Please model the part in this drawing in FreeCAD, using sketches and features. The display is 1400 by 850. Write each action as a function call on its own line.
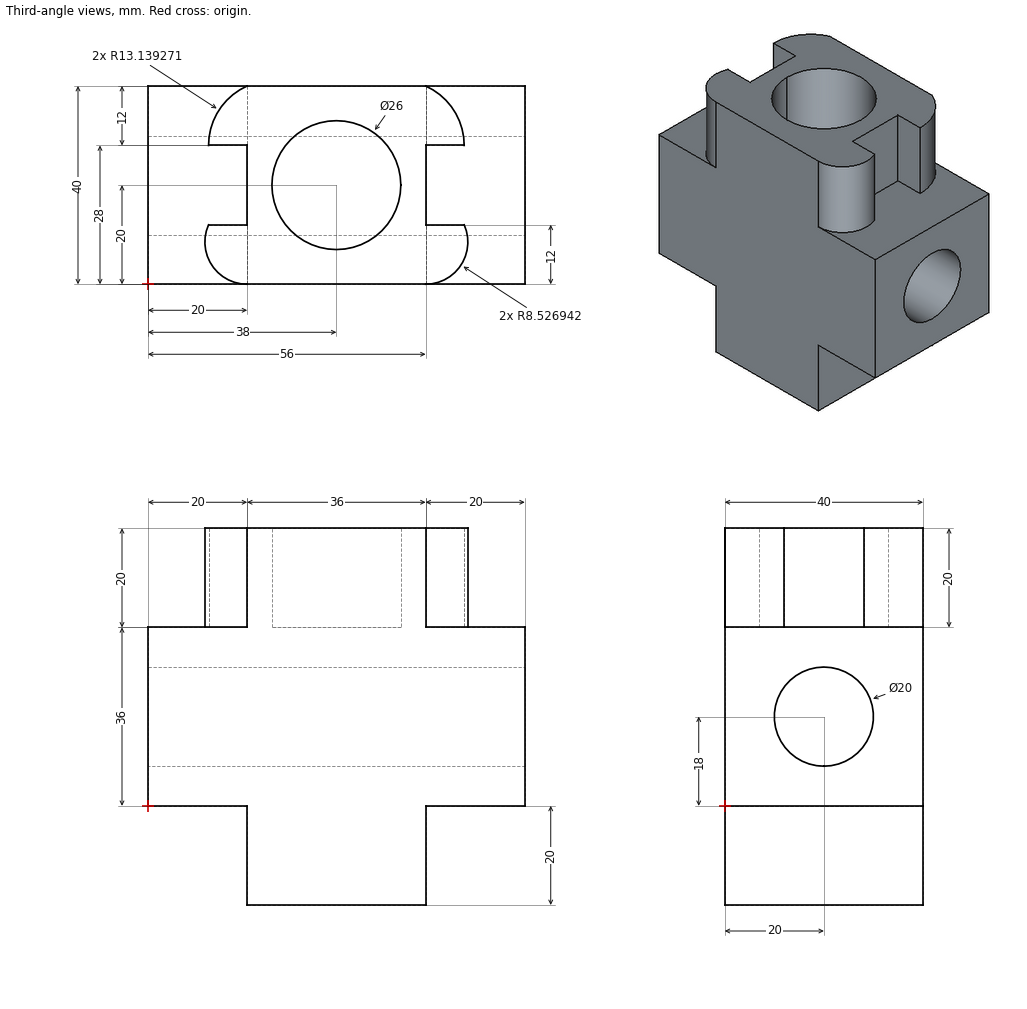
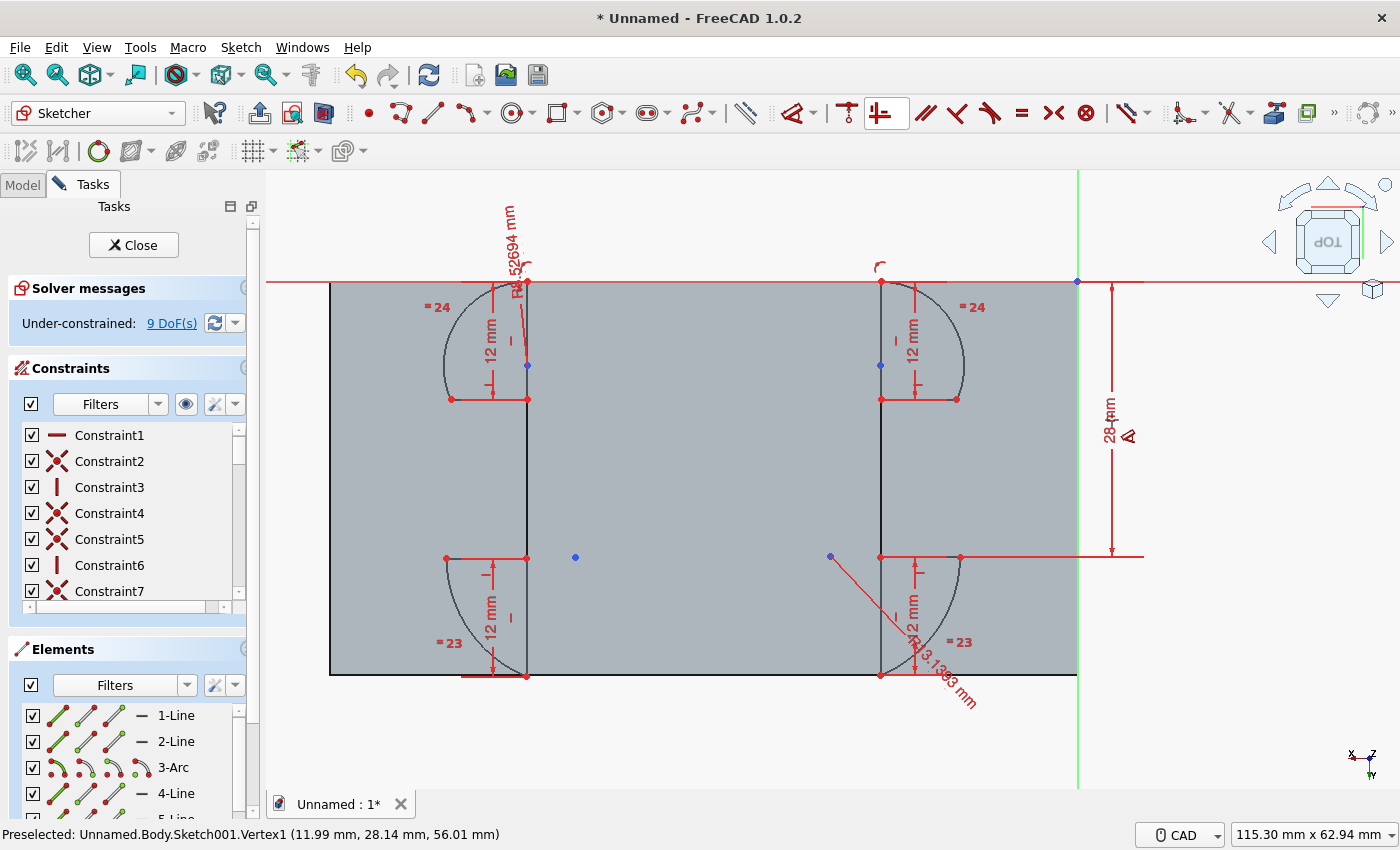
click(881, 557)
click(979, 248)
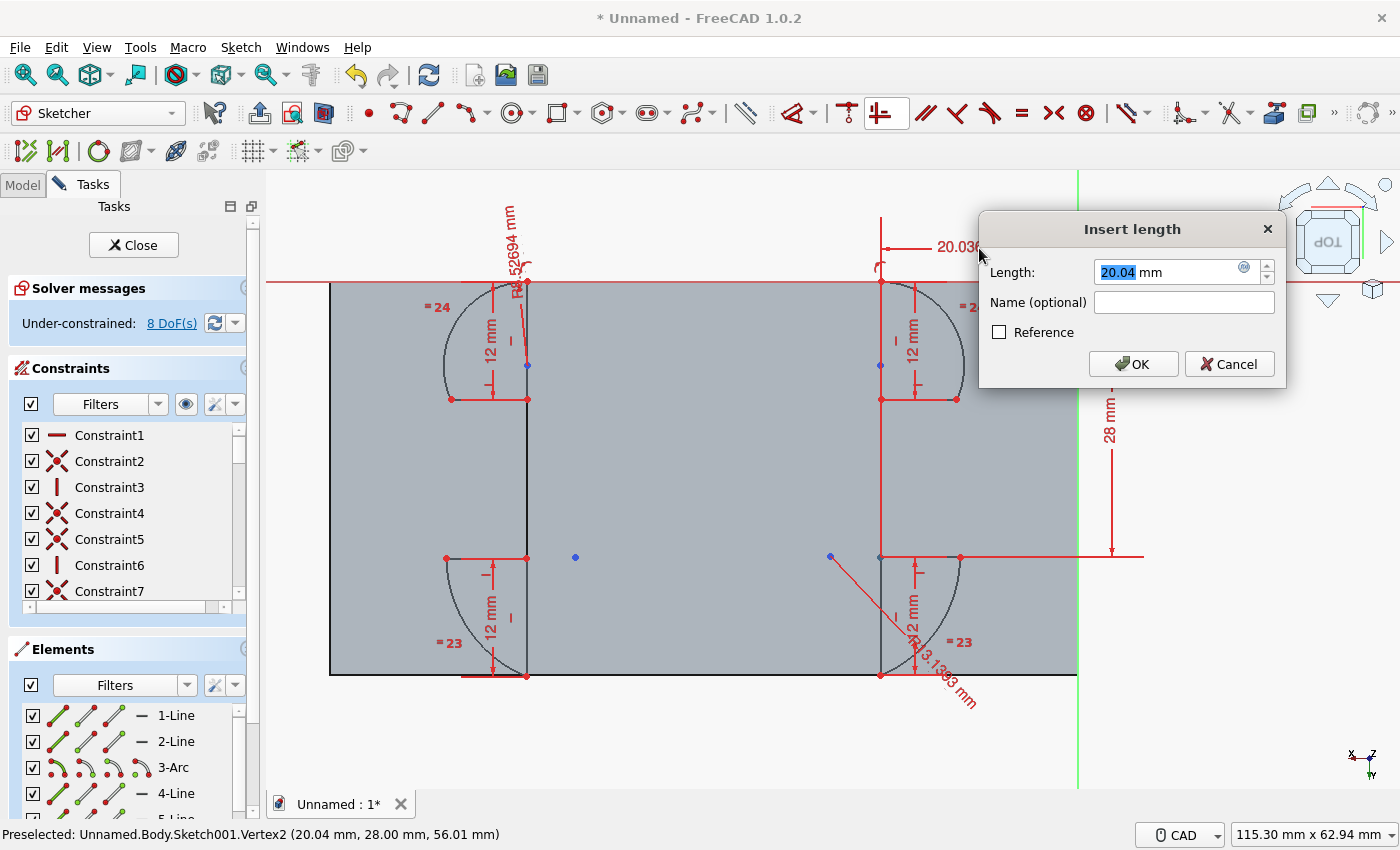
text(20)
key(Return)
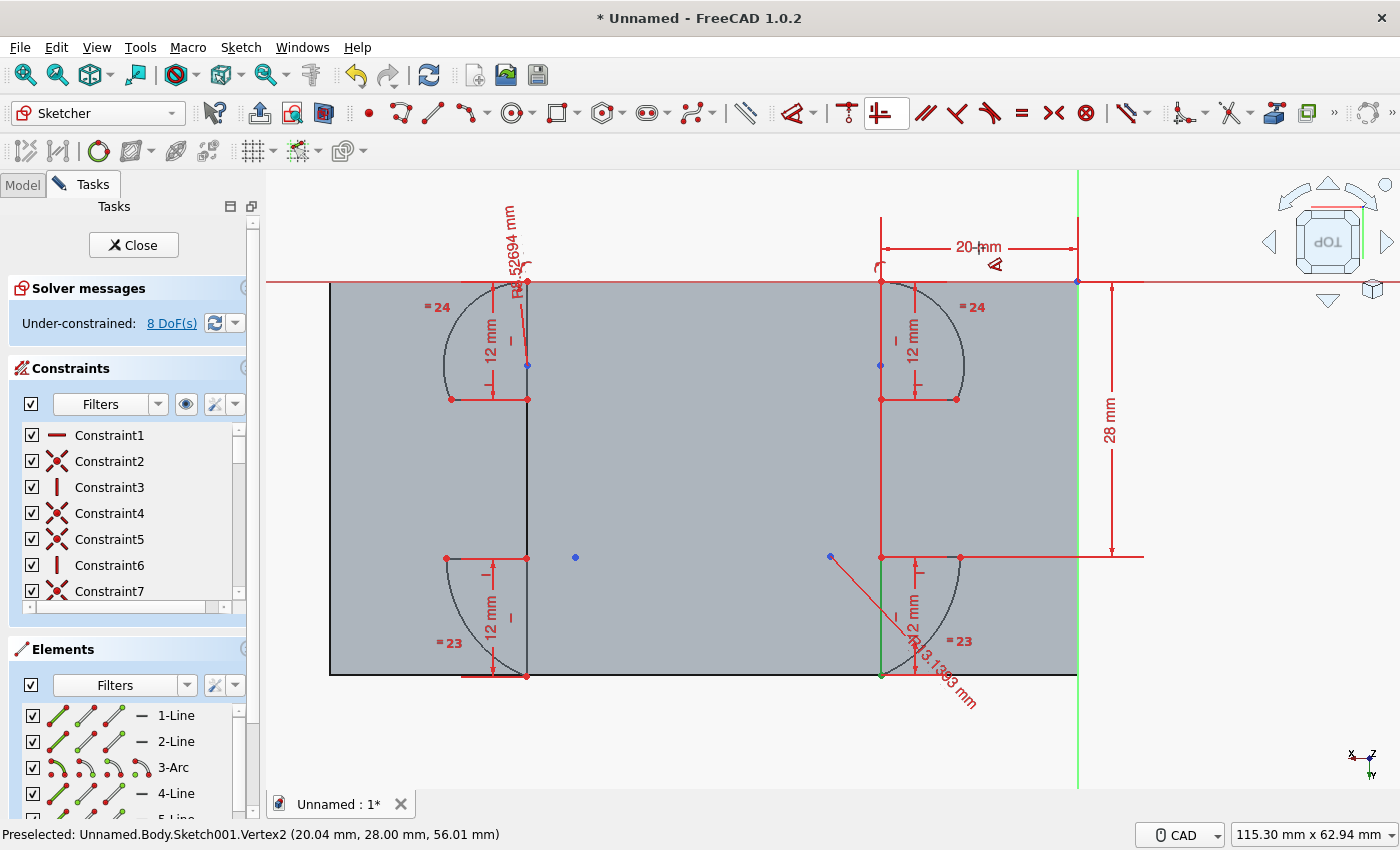
click(527, 677)
click(802, 711)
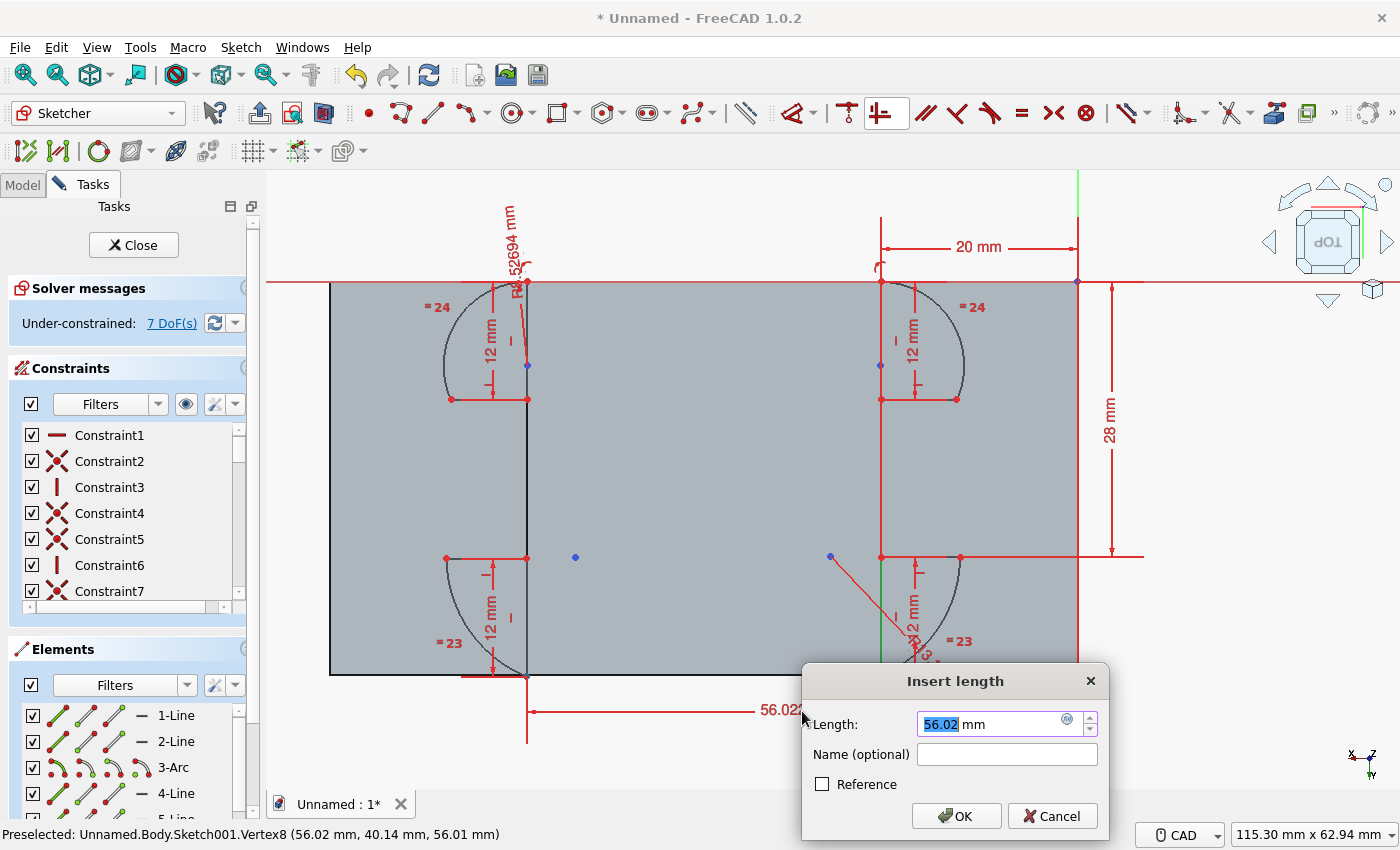
text(56)
key(Return)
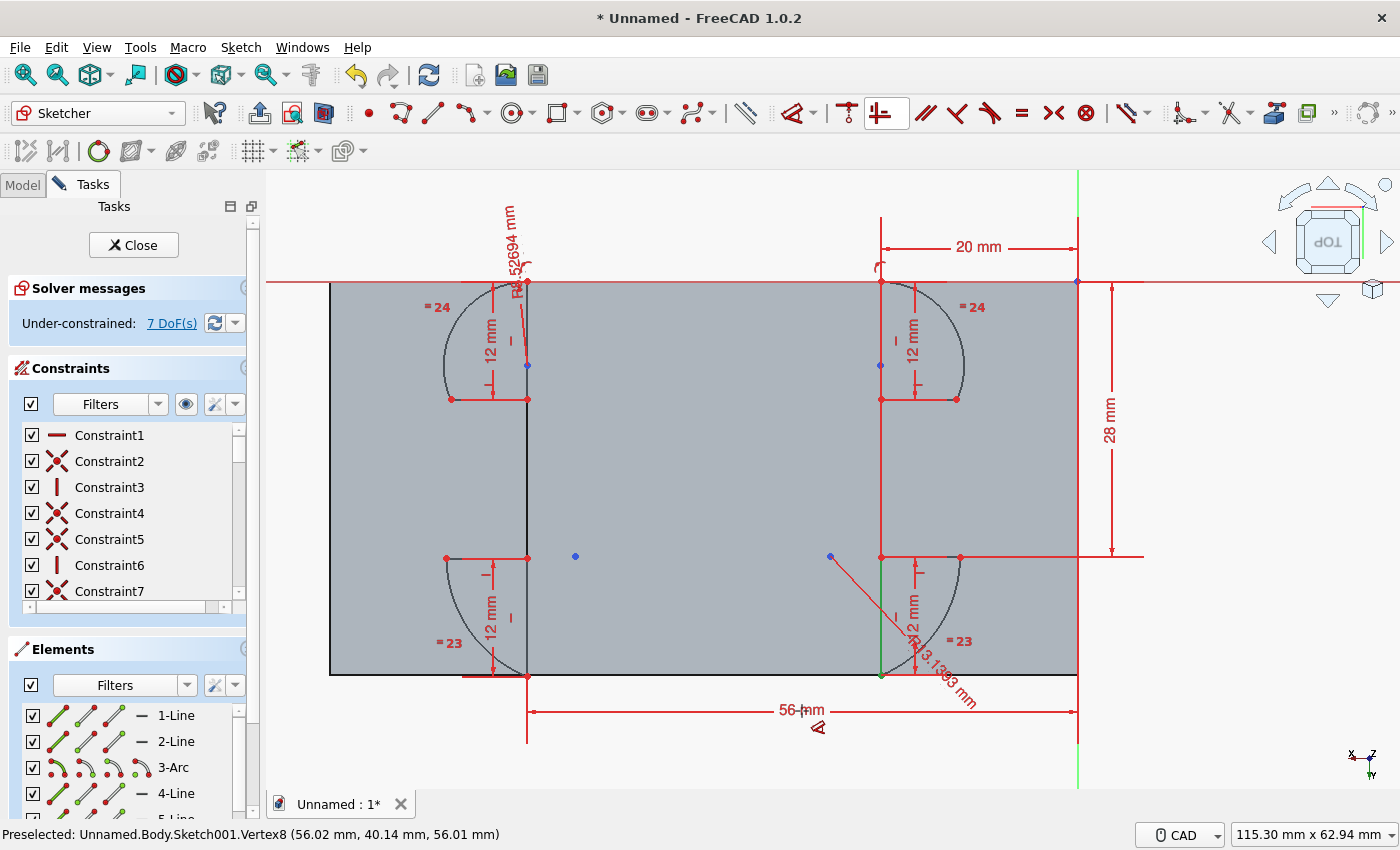
click(527, 677)
click(1112, 479)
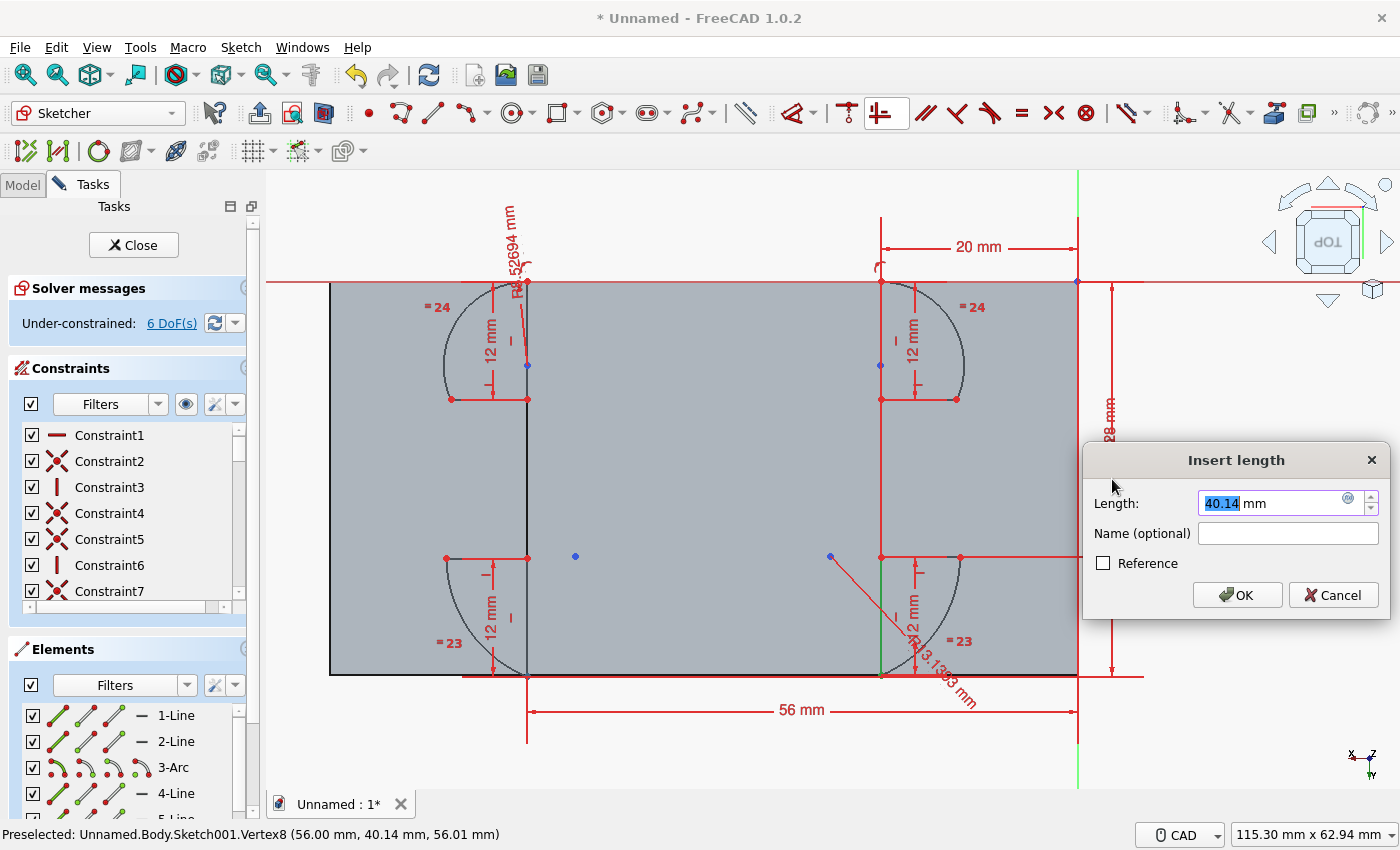
text(40)
key(Return)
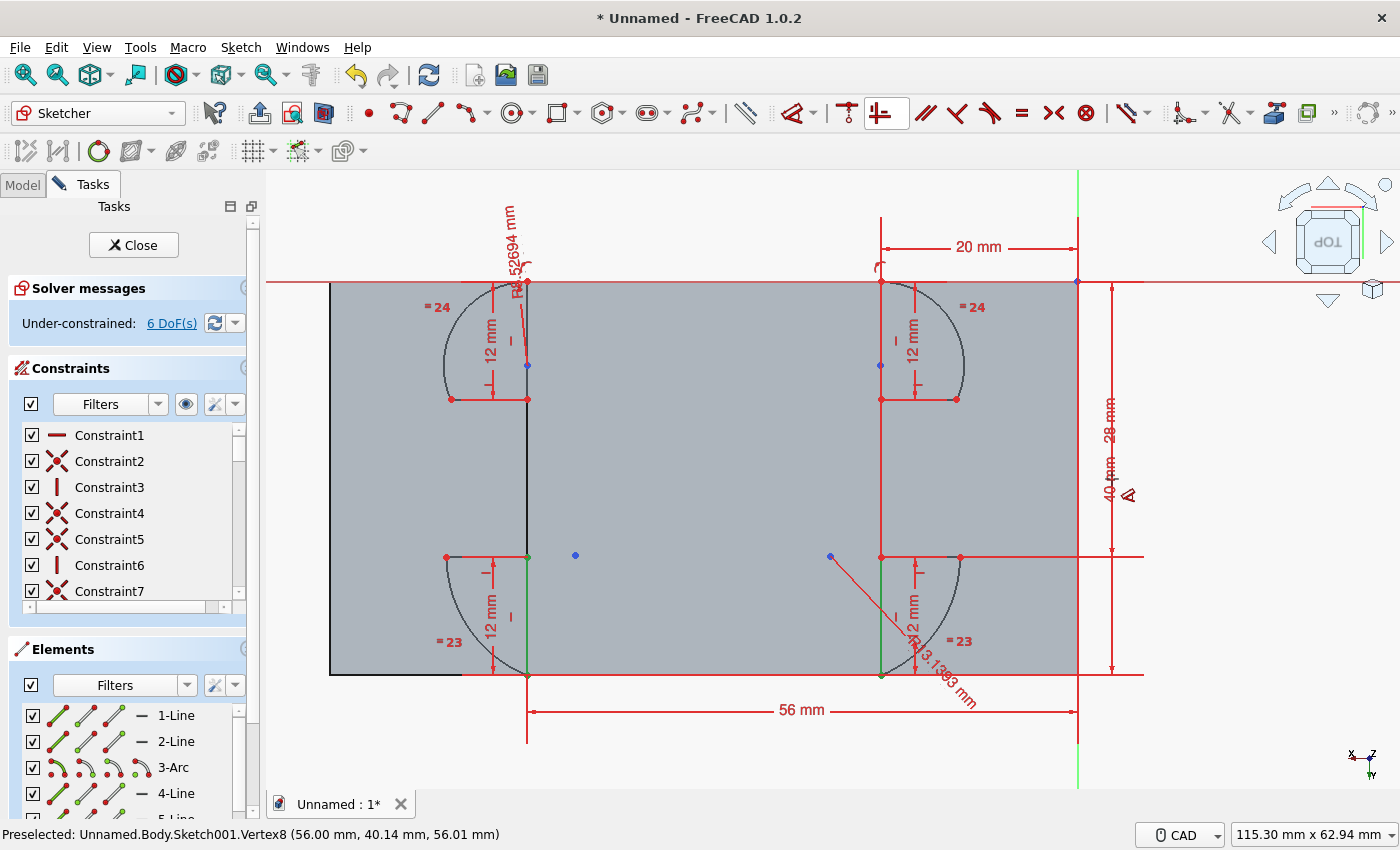
click(527, 400)
click(802, 248)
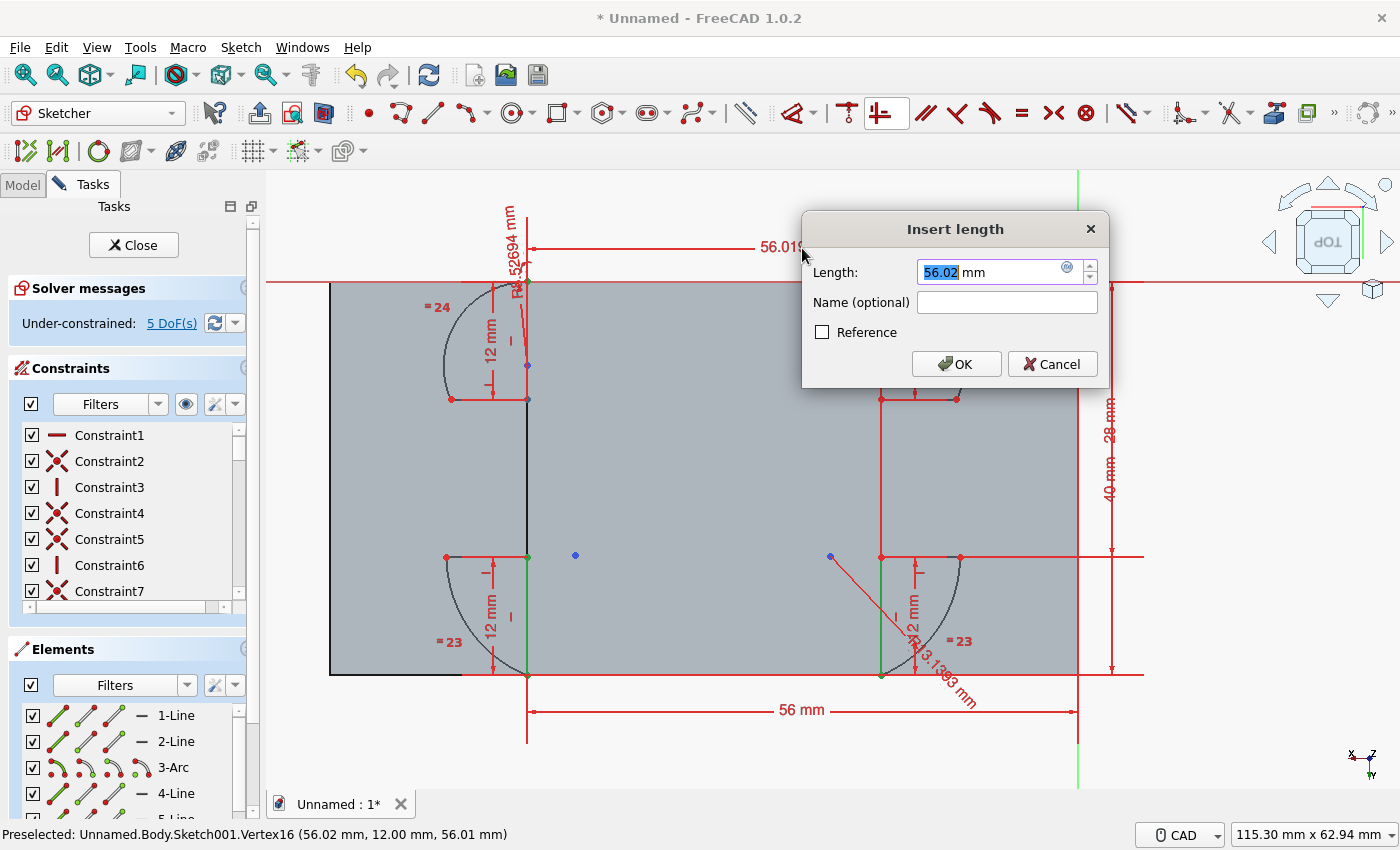
text(56)
key(Return)